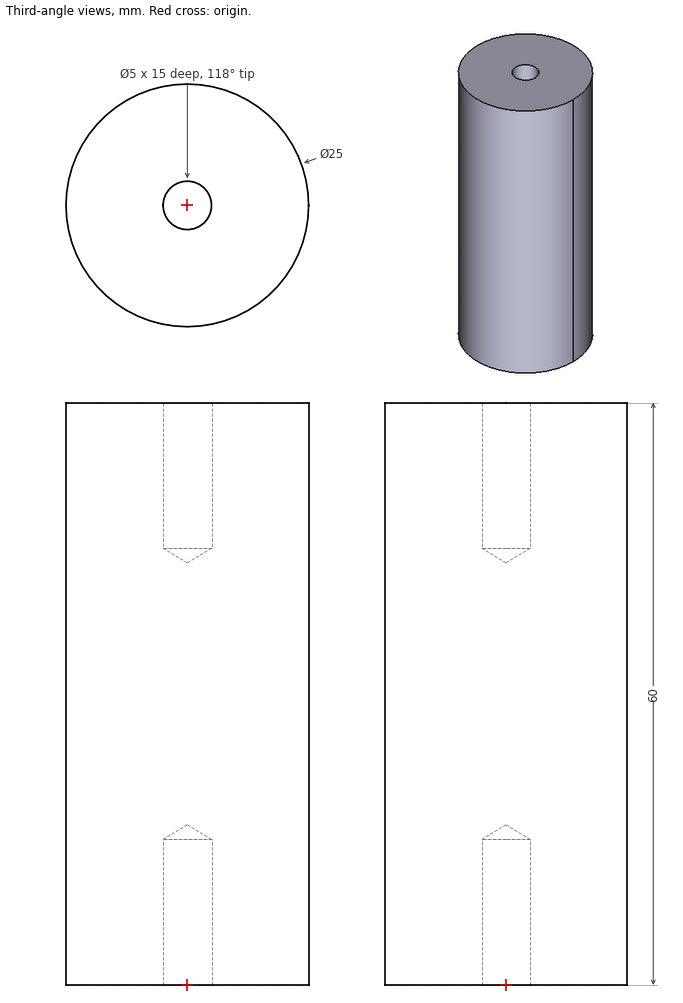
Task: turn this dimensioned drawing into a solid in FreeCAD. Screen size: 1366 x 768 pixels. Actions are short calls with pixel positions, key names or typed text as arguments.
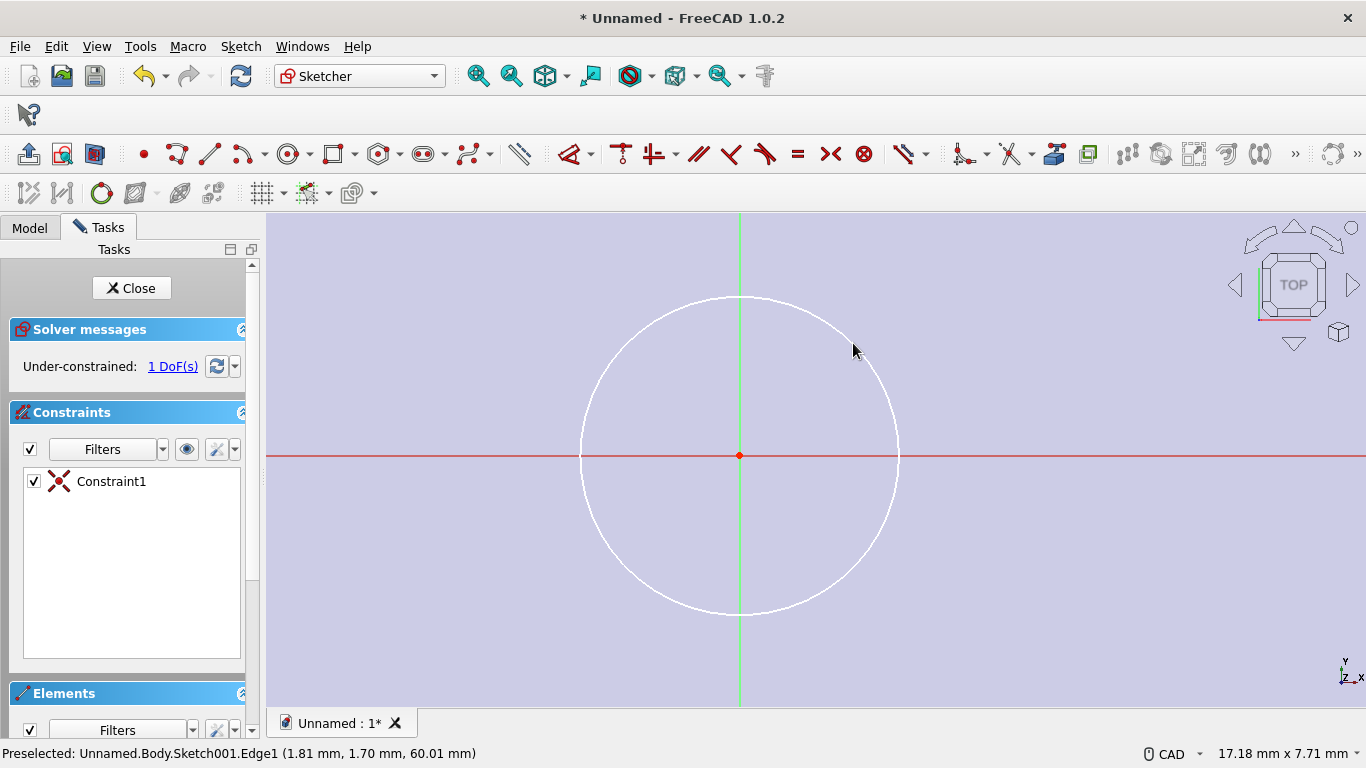
click(568, 154)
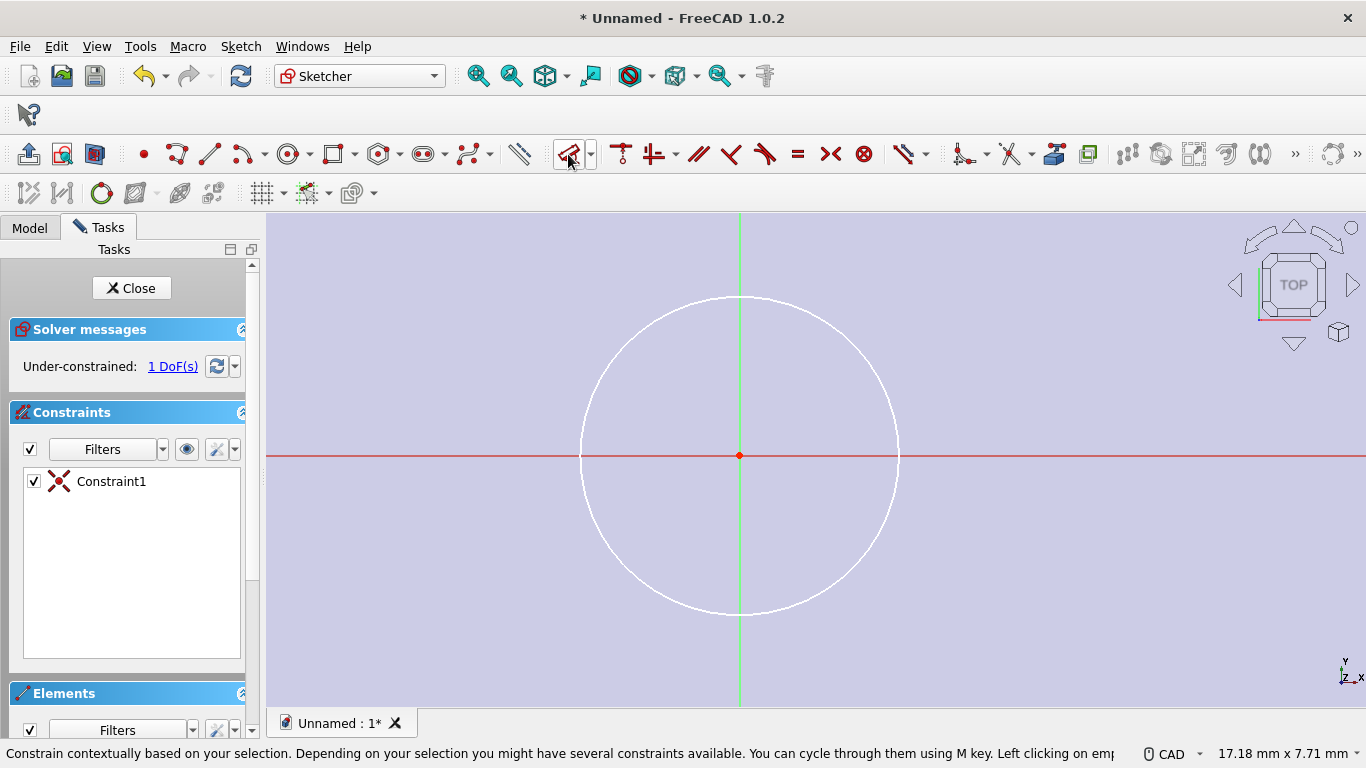
click(852, 343)
click(875, 320)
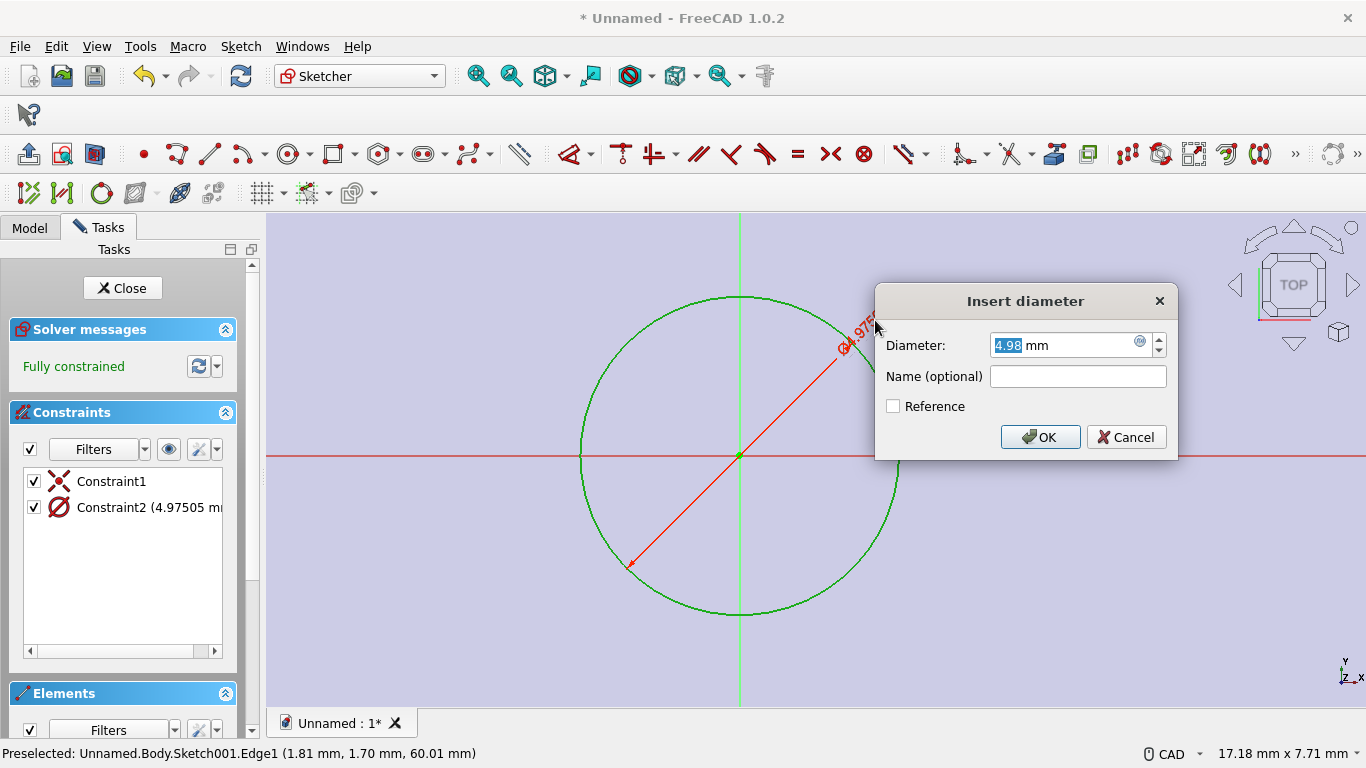
text(5)
key(Return)
key(Escape)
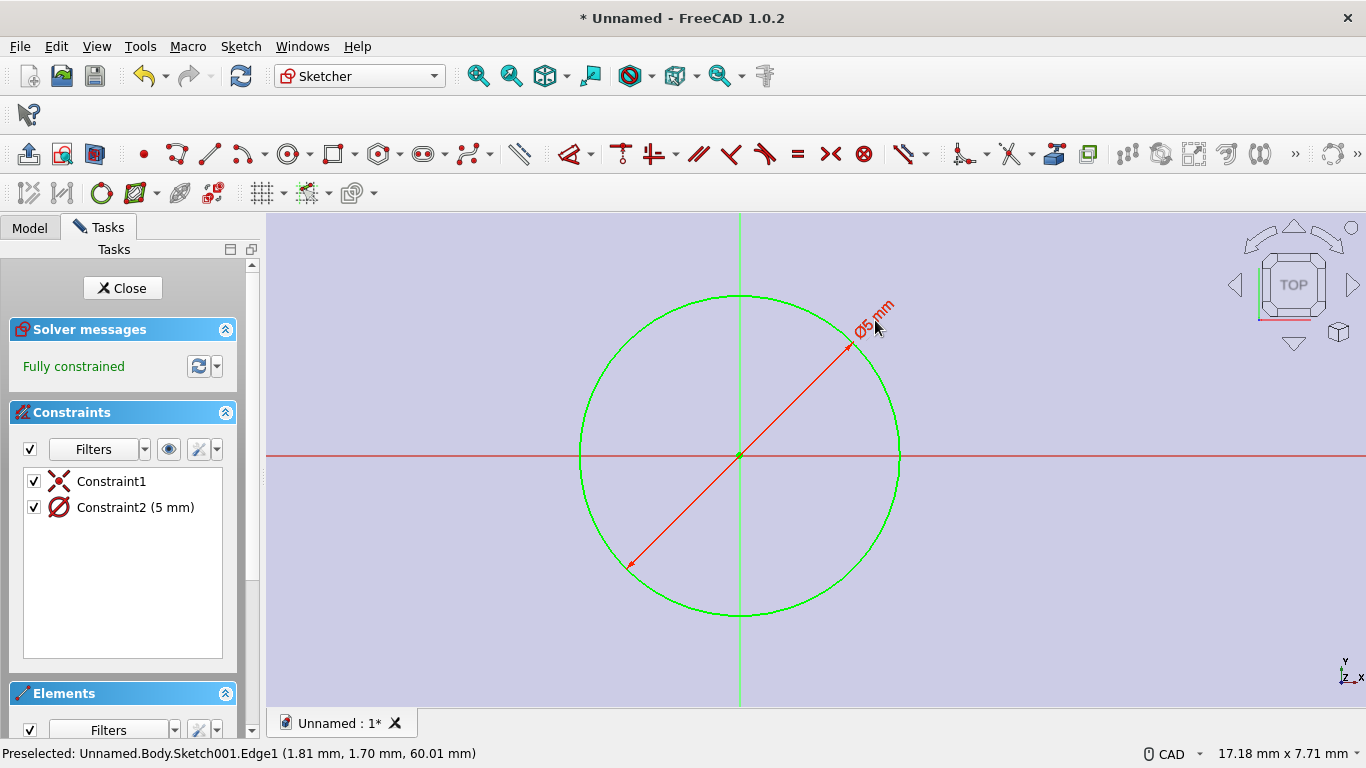
click(123, 288)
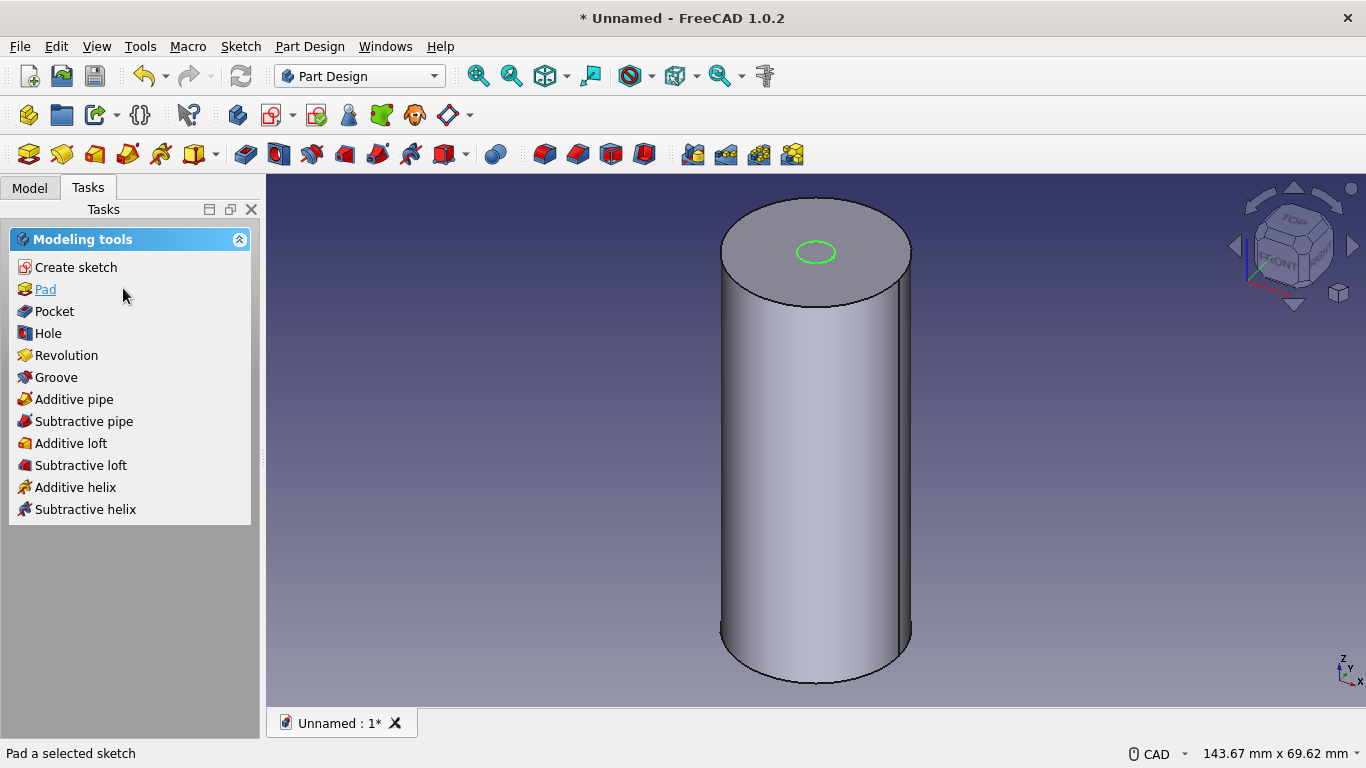
click(279, 154)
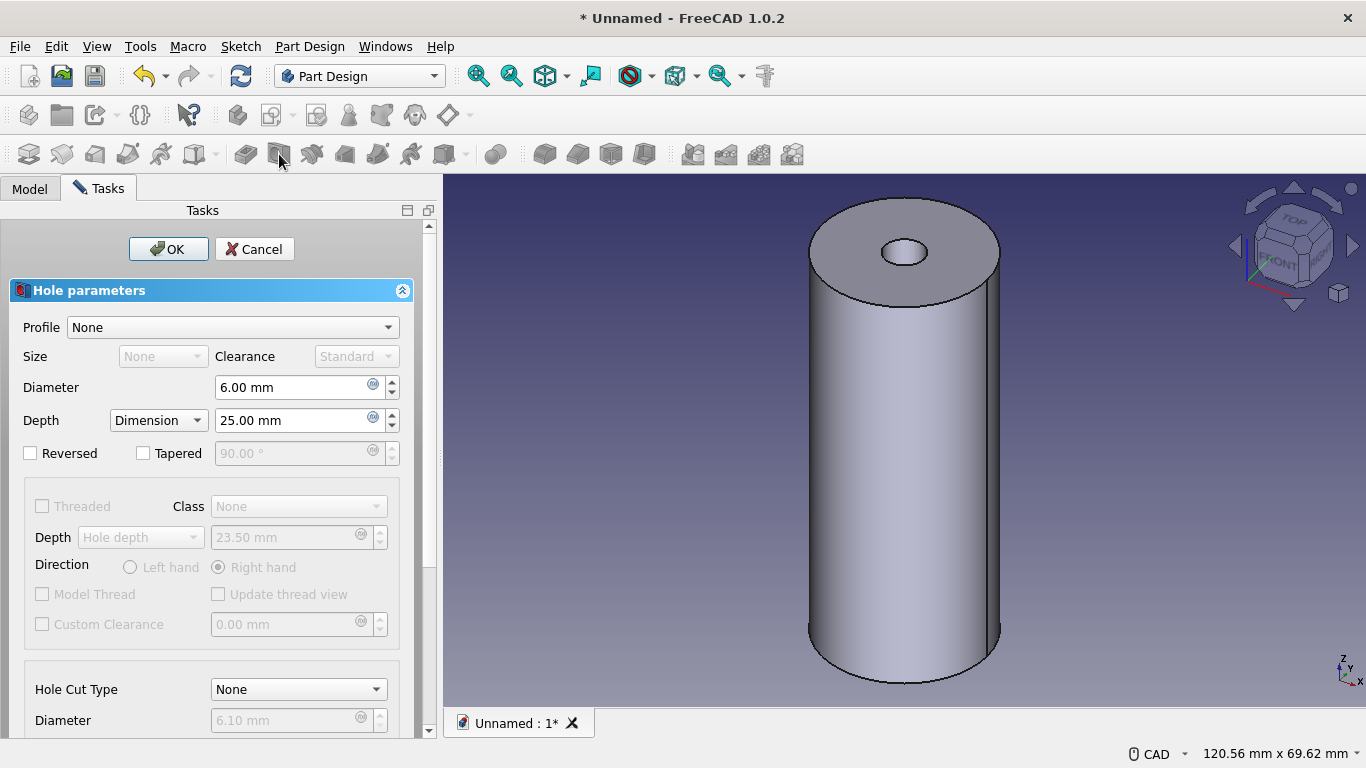
triple_click(300, 388)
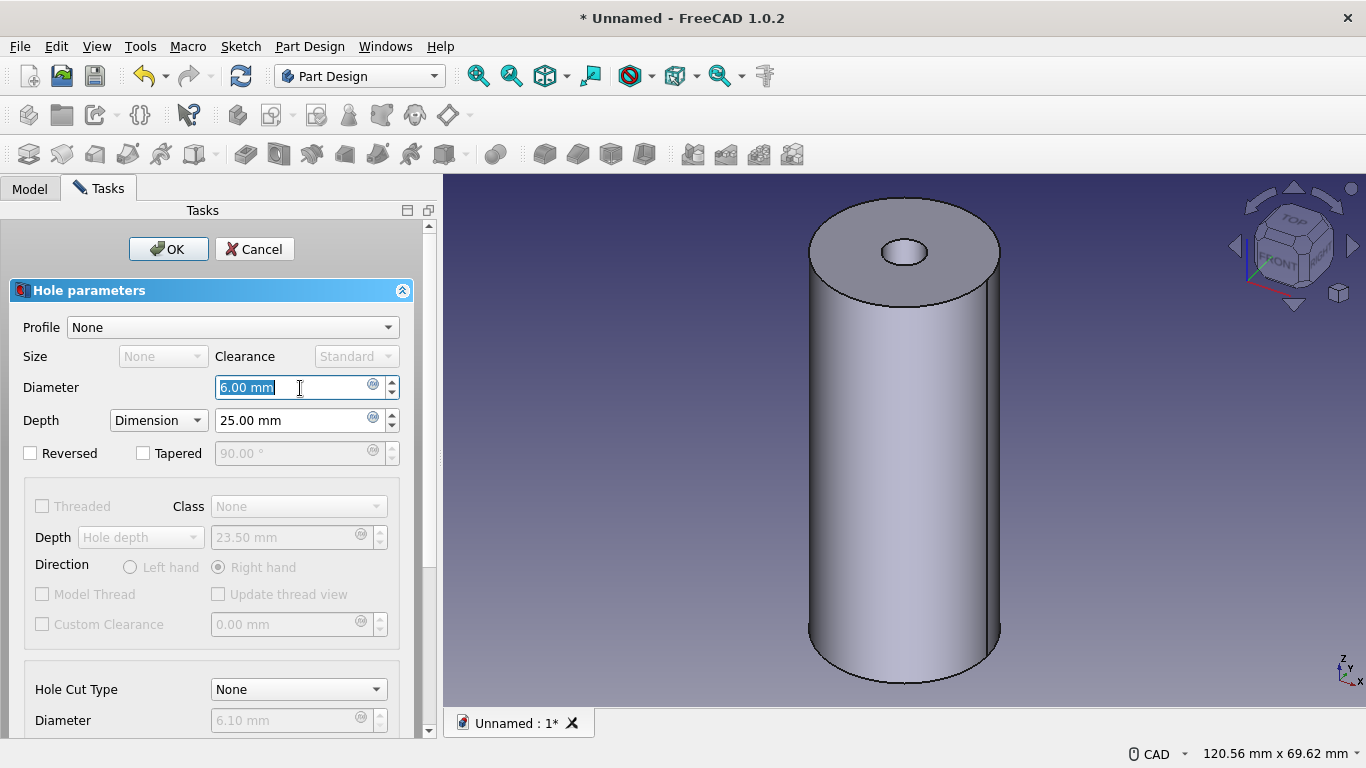
text(5)
key(Tab)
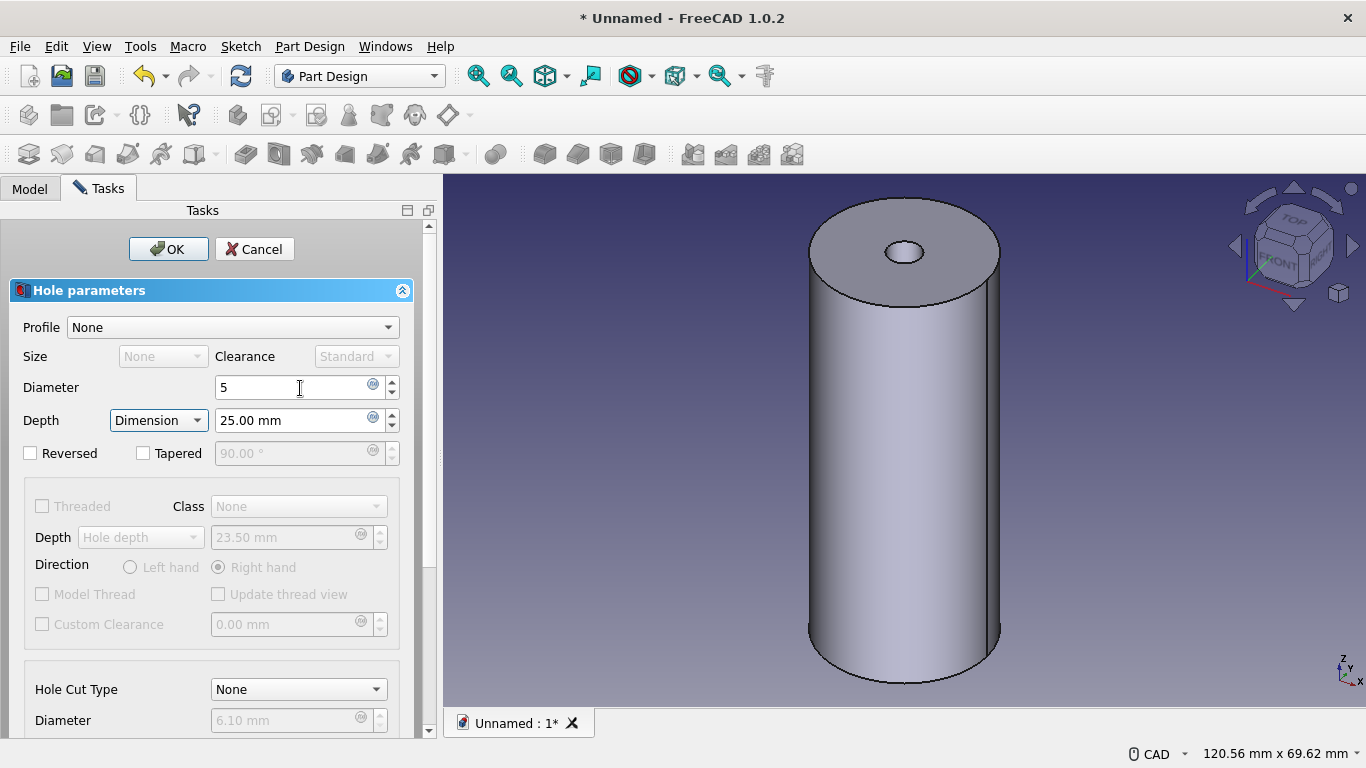
triple_click(300, 420)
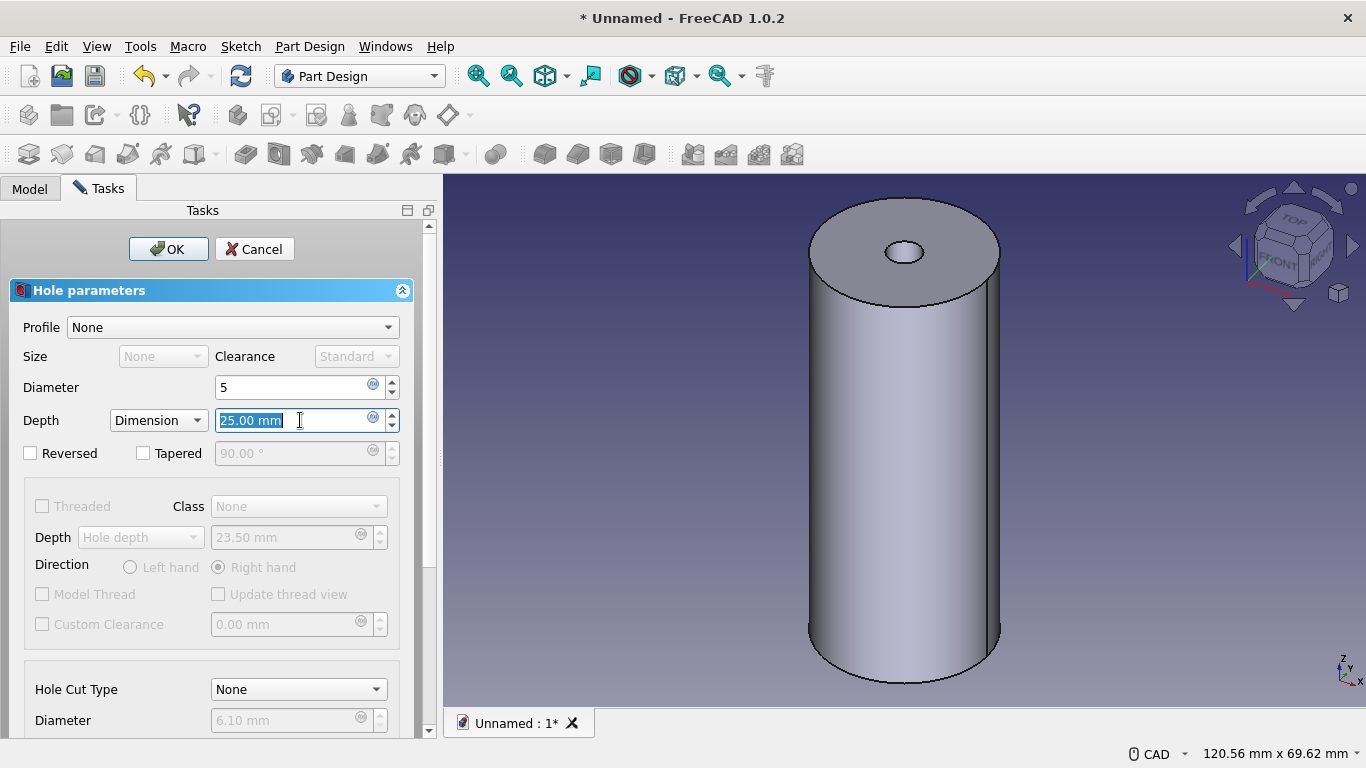
text(15)
key(Tab)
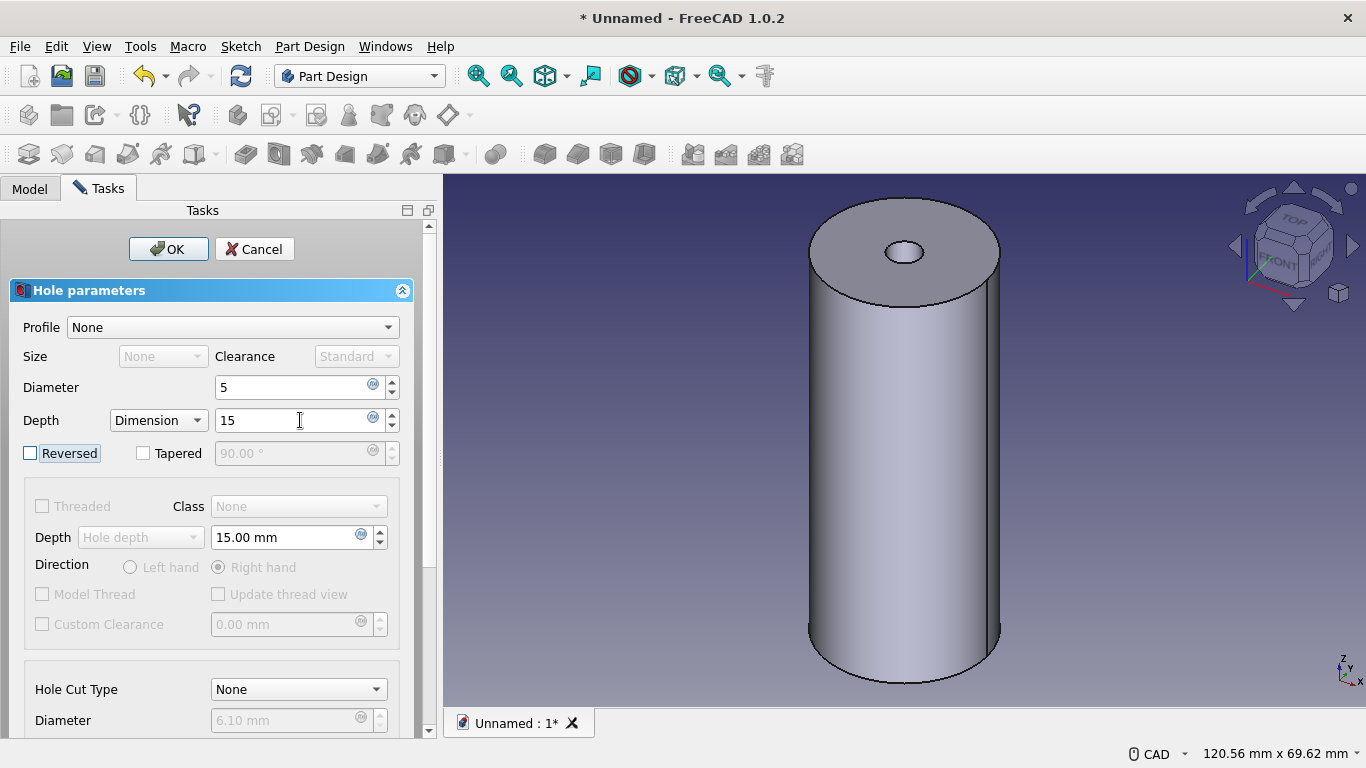
click(169, 249)